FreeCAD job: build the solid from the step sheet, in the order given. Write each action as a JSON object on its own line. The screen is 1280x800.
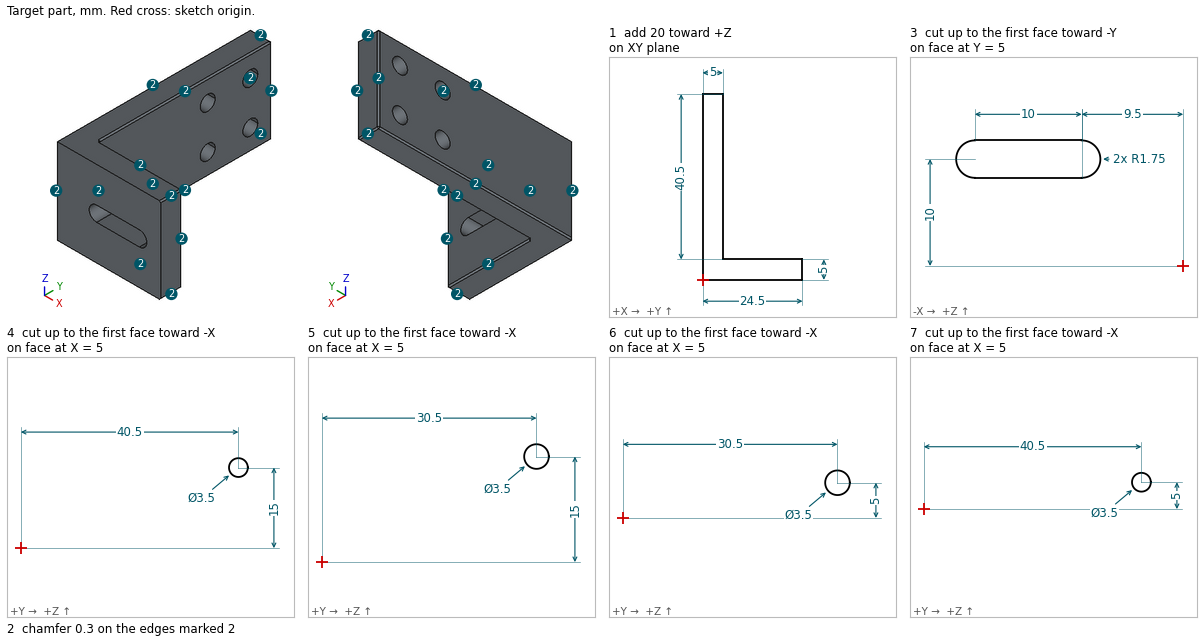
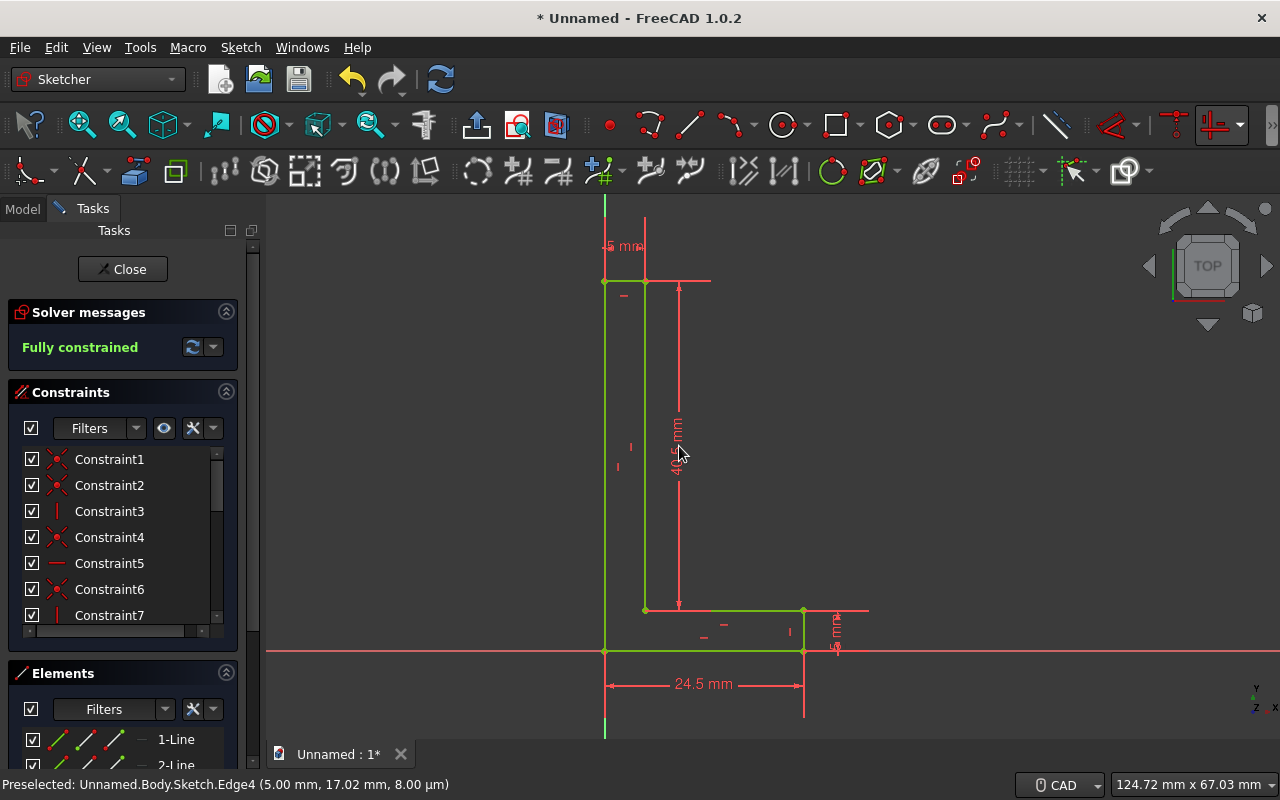
{"action": "left_click", "coordinate": [123, 269]}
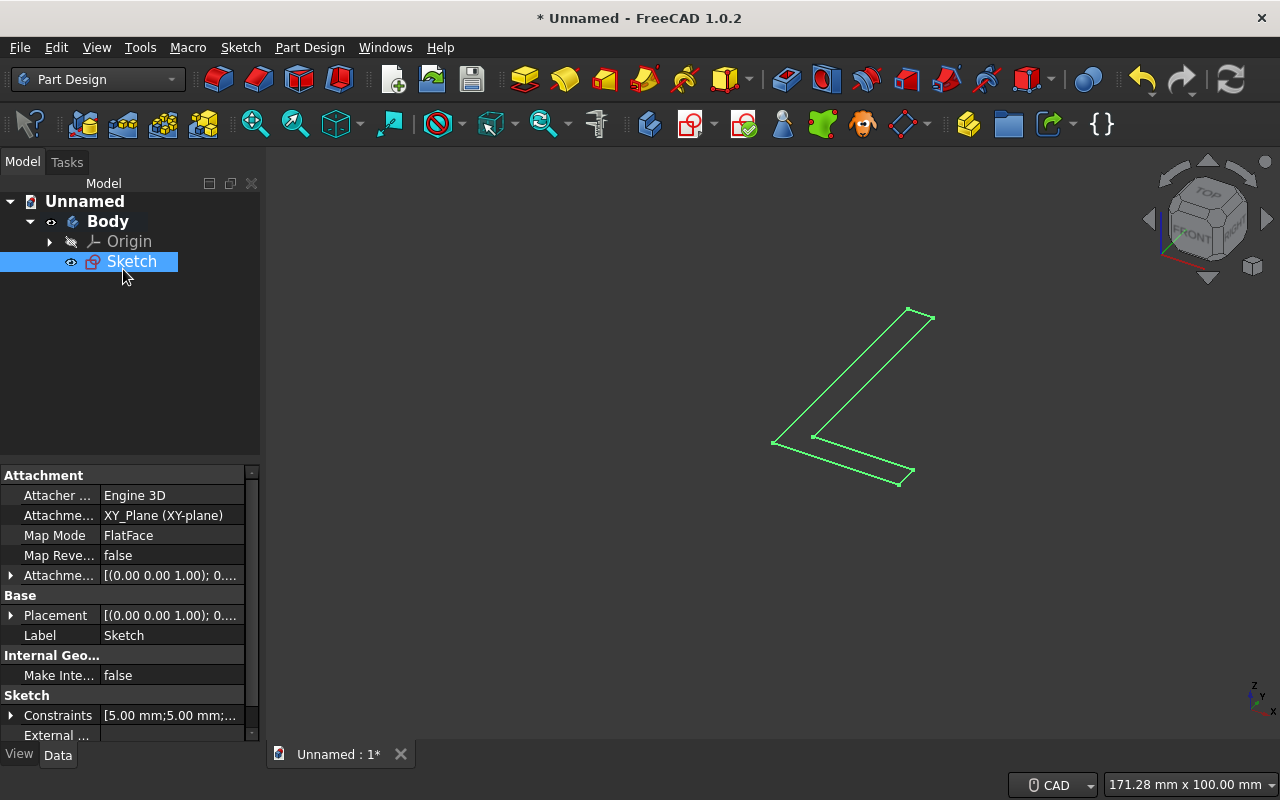
{"action": "left_click", "coordinate": [526, 80]}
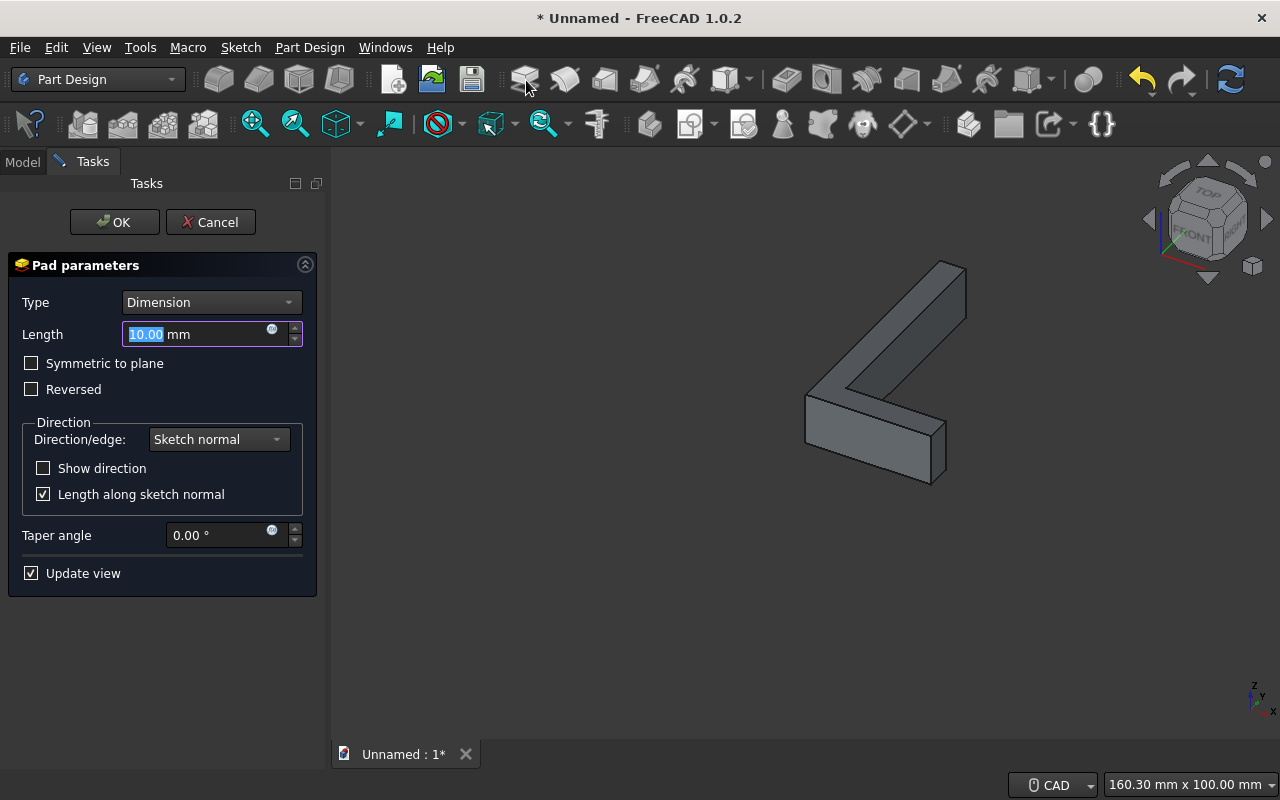
{"action": "type", "text": "20"}
{"action": "key", "text": "Tab"}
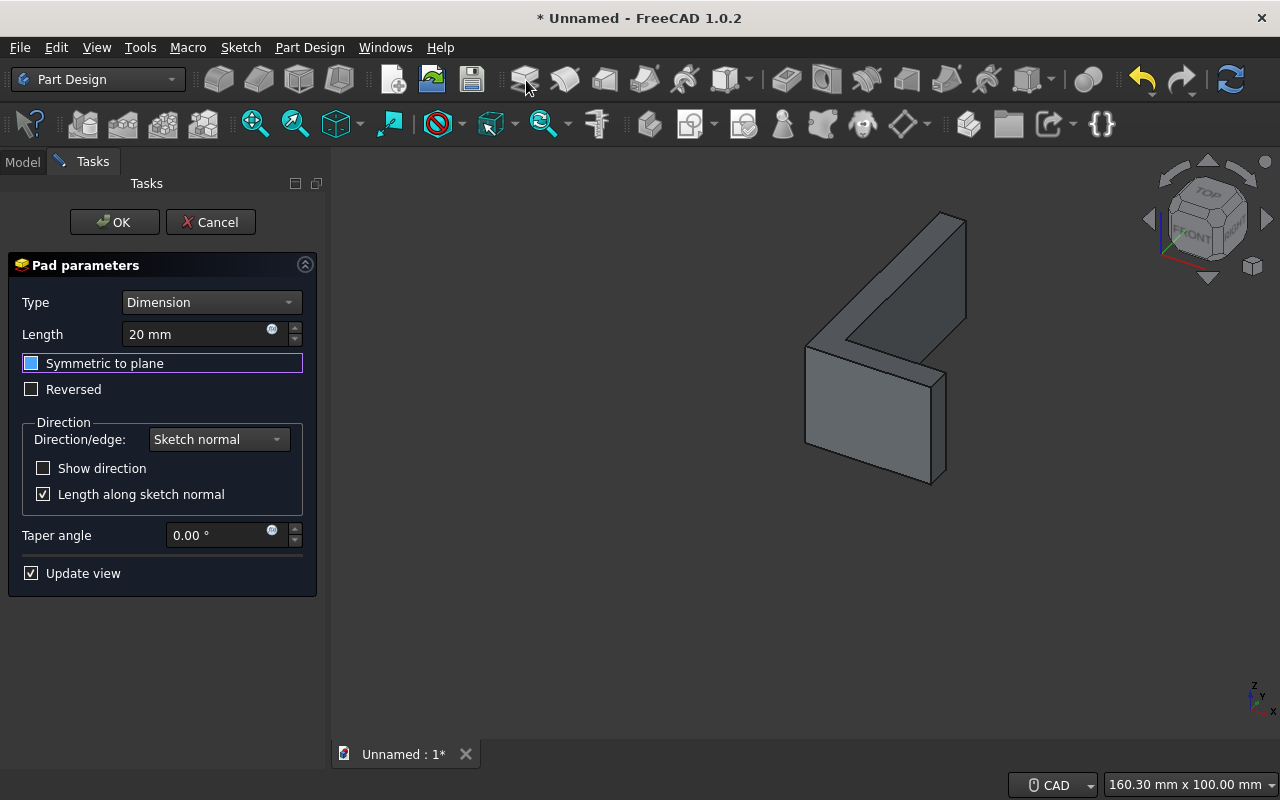
{"action": "left_click", "coordinate": [115, 222]}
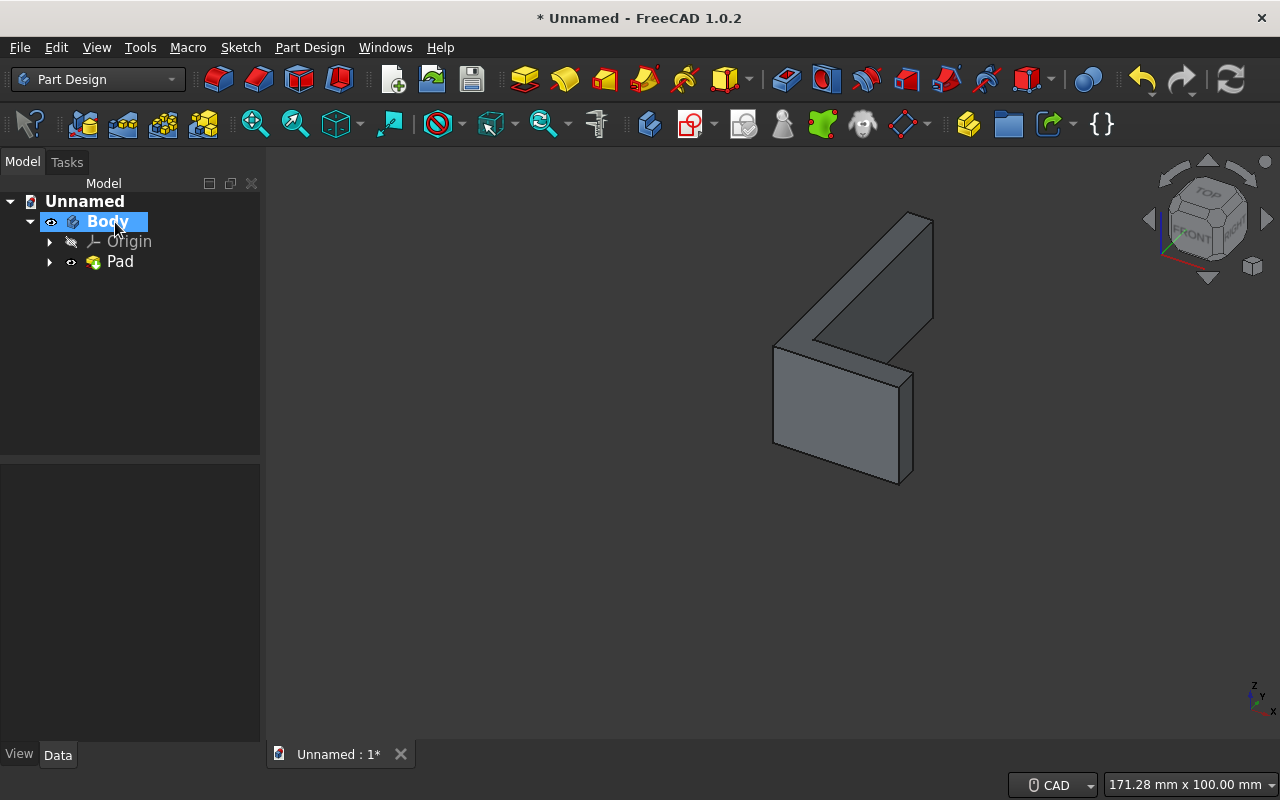
{"action": "left_click", "coordinate": [890, 311]}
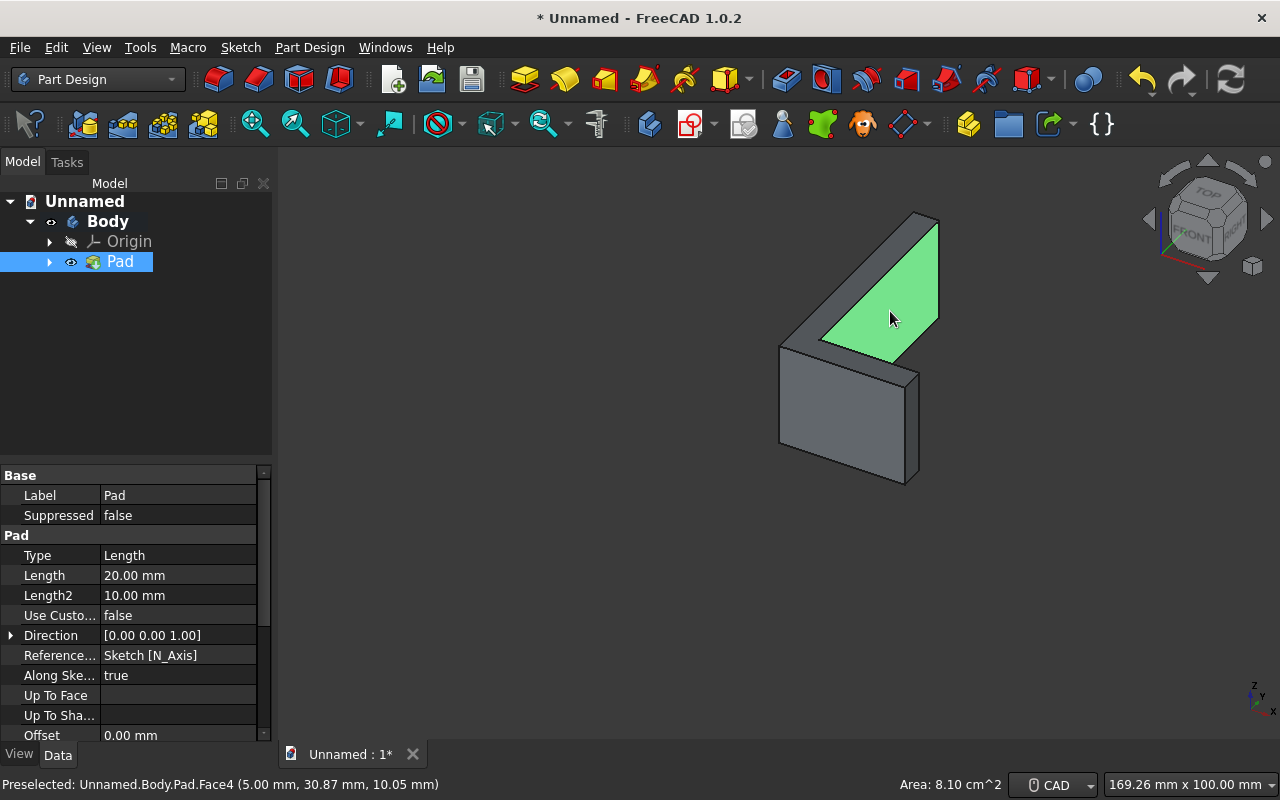
{"action": "left_click", "coordinate": [912, 379], "text": "ctrl"}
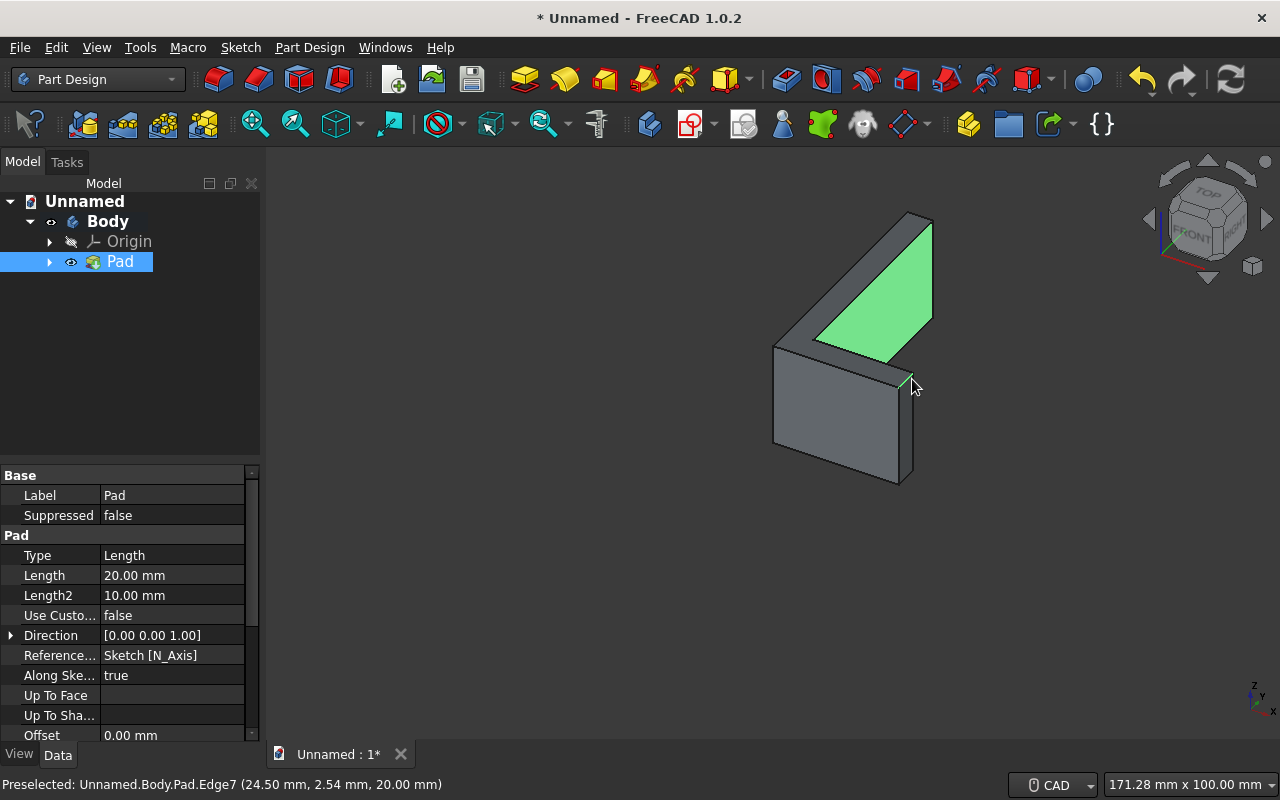
{"action": "key", "text": "0"}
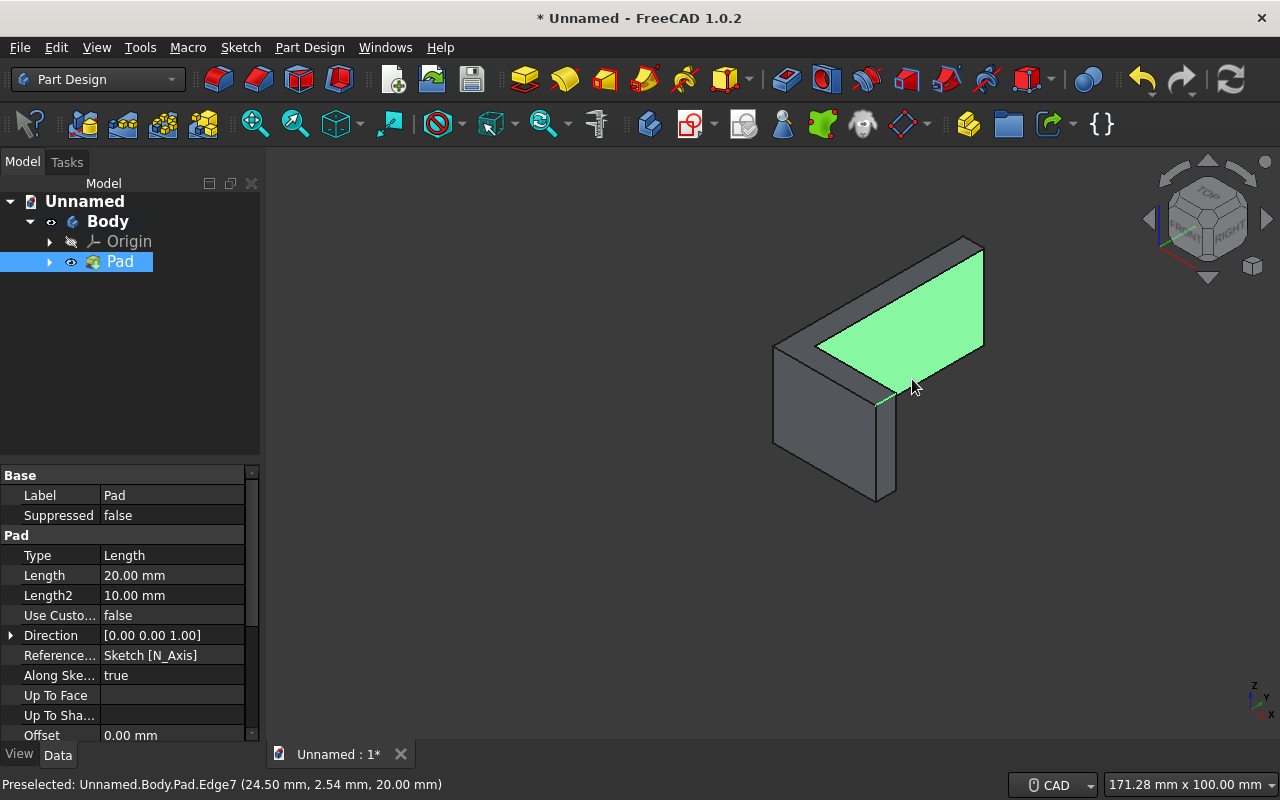
{"action": "left_click", "coordinate": [256, 124]}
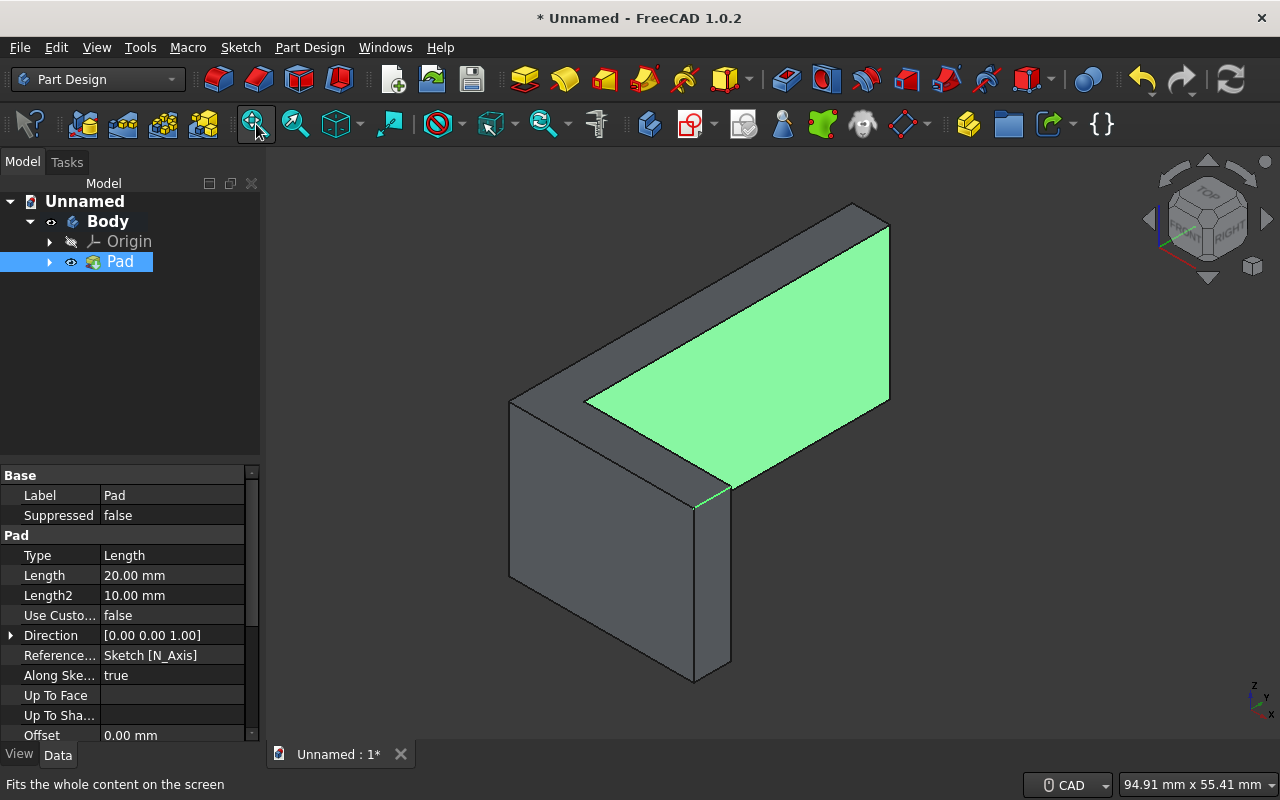
{"action": "key", "text": "2"}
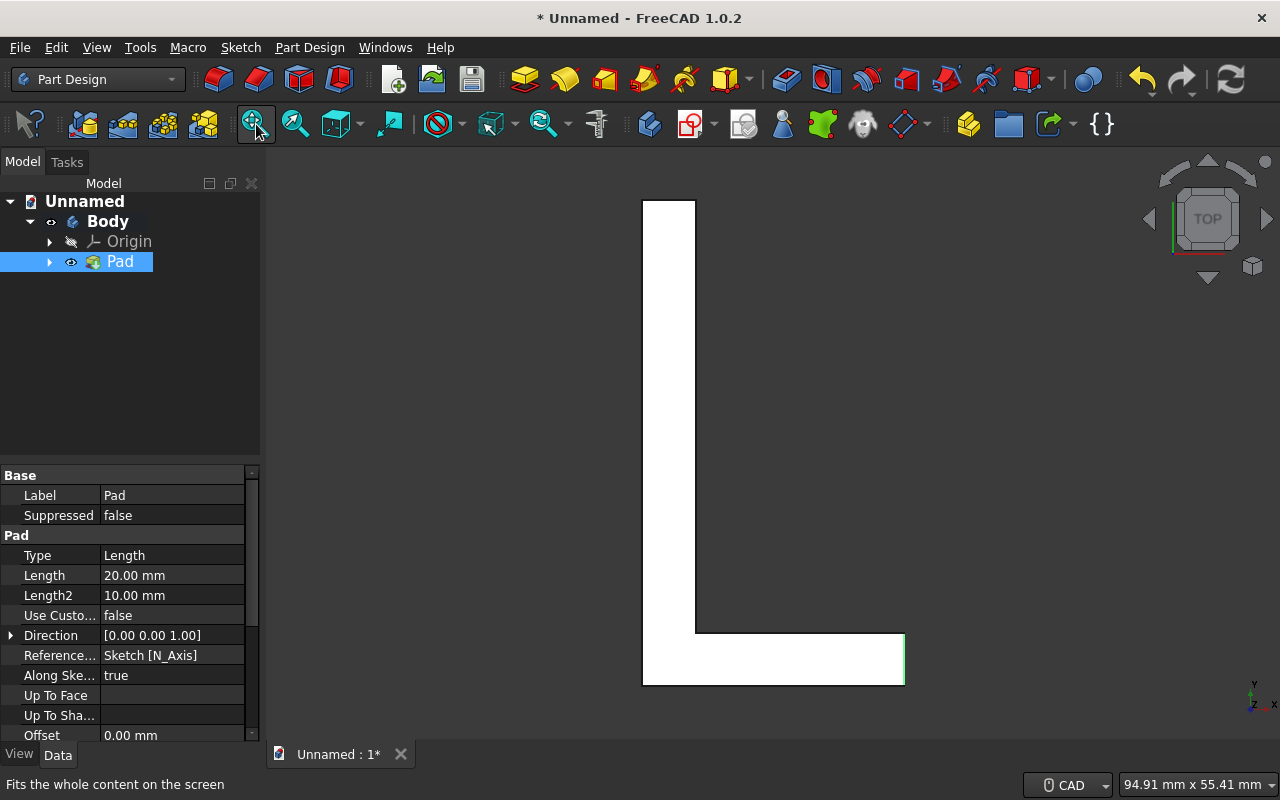
{"action": "left_click", "coordinate": [669, 199], "text": "ctrl"}